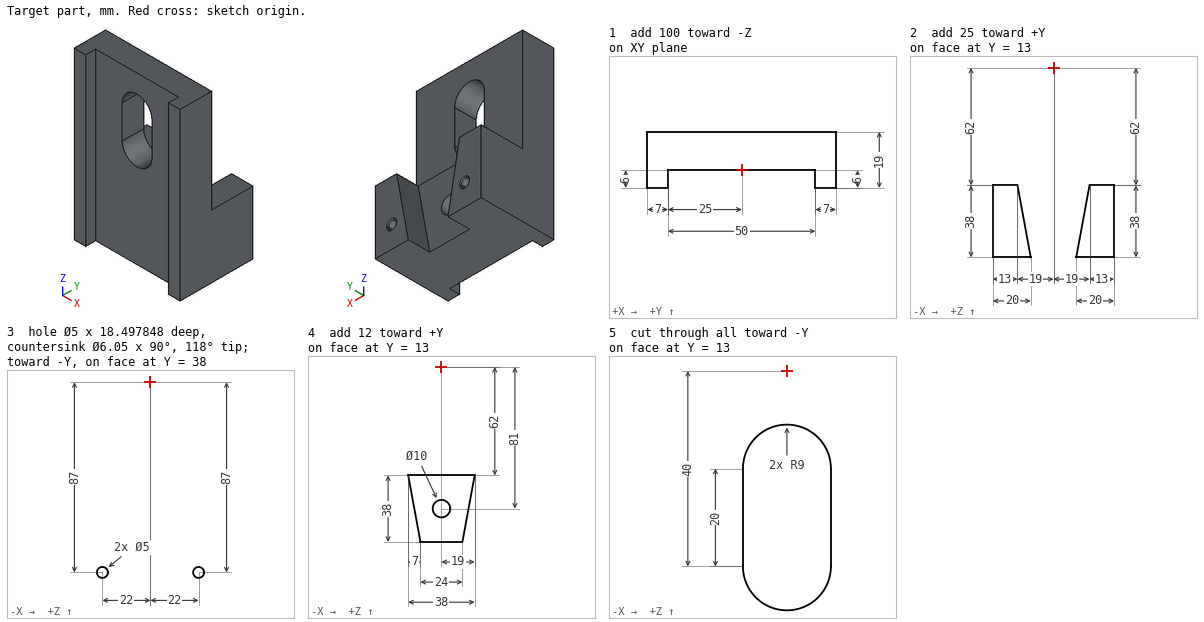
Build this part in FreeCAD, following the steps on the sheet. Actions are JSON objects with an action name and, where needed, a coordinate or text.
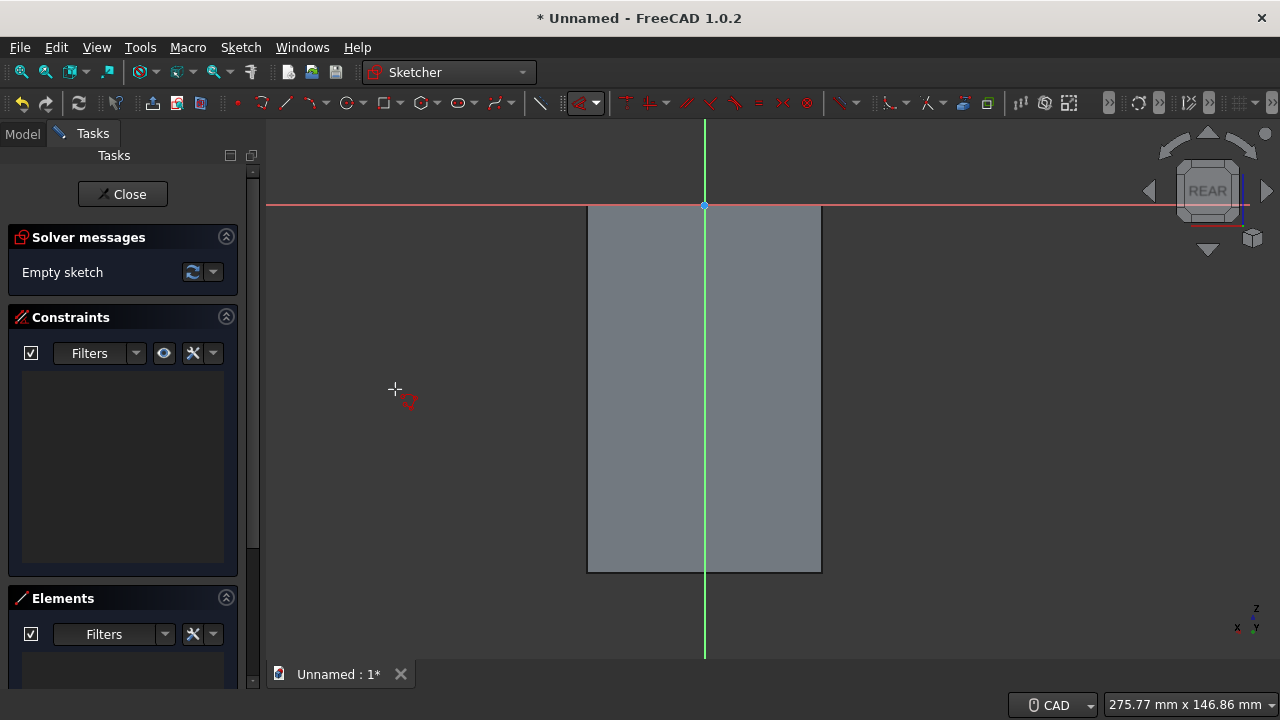
{"action": "left_click", "coordinate": [635, 433]}
{"action": "left_click", "coordinate": [587, 433]}
{"action": "left_click", "coordinate": [587, 573]}
{"action": "left_click", "coordinate": [660, 573]}
{"action": "left_click", "coordinate": [635, 434]}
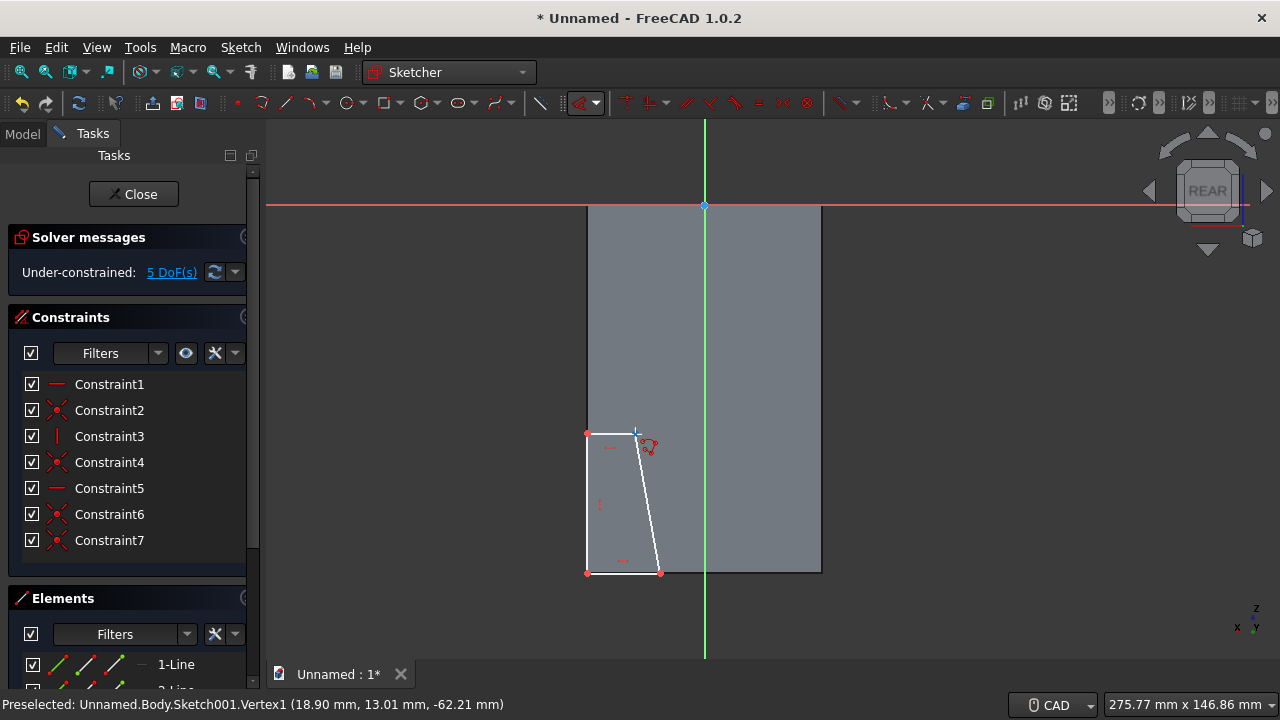
{"action": "left_click", "coordinate": [774, 433]}
{"action": "left_click", "coordinate": [749, 573]}
{"action": "left_click", "coordinate": [822, 573]}
{"action": "left_click", "coordinate": [822, 433]}
{"action": "left_click", "coordinate": [774, 434]}
{"action": "key", "text": "Escape"}
{"action": "key", "text": "Escape"}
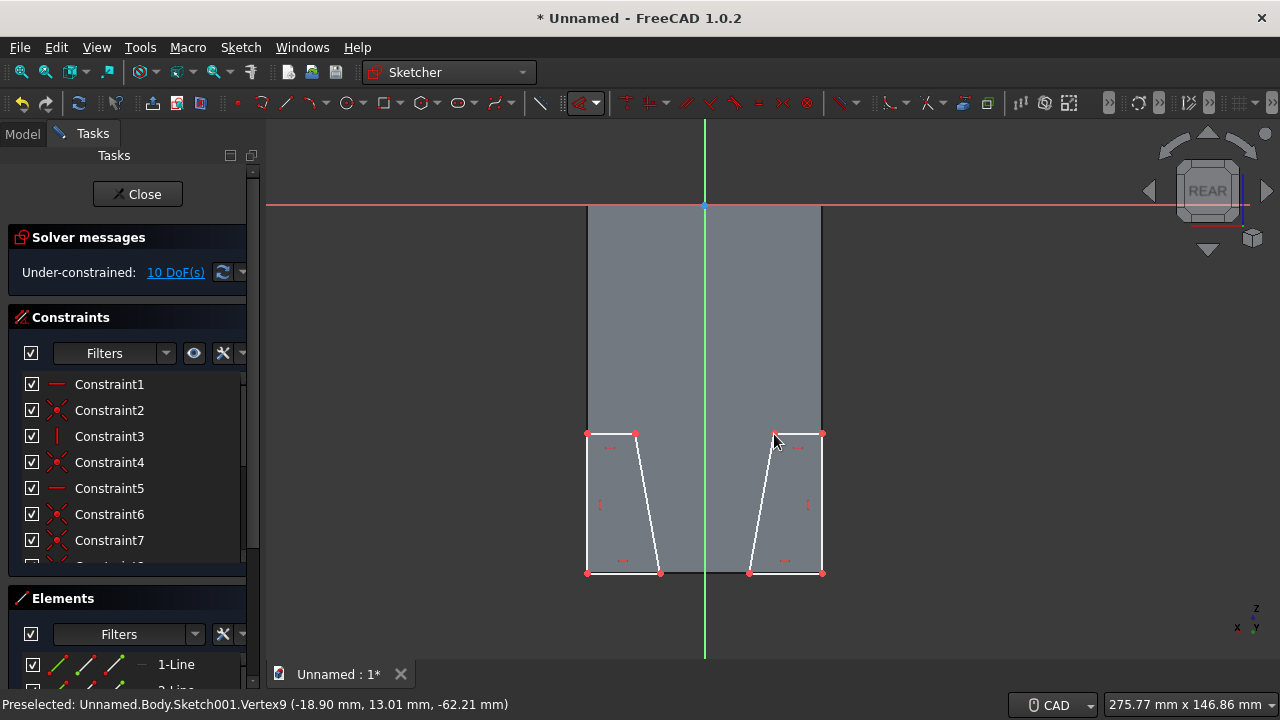
{"action": "left_click", "coordinate": [580, 104]}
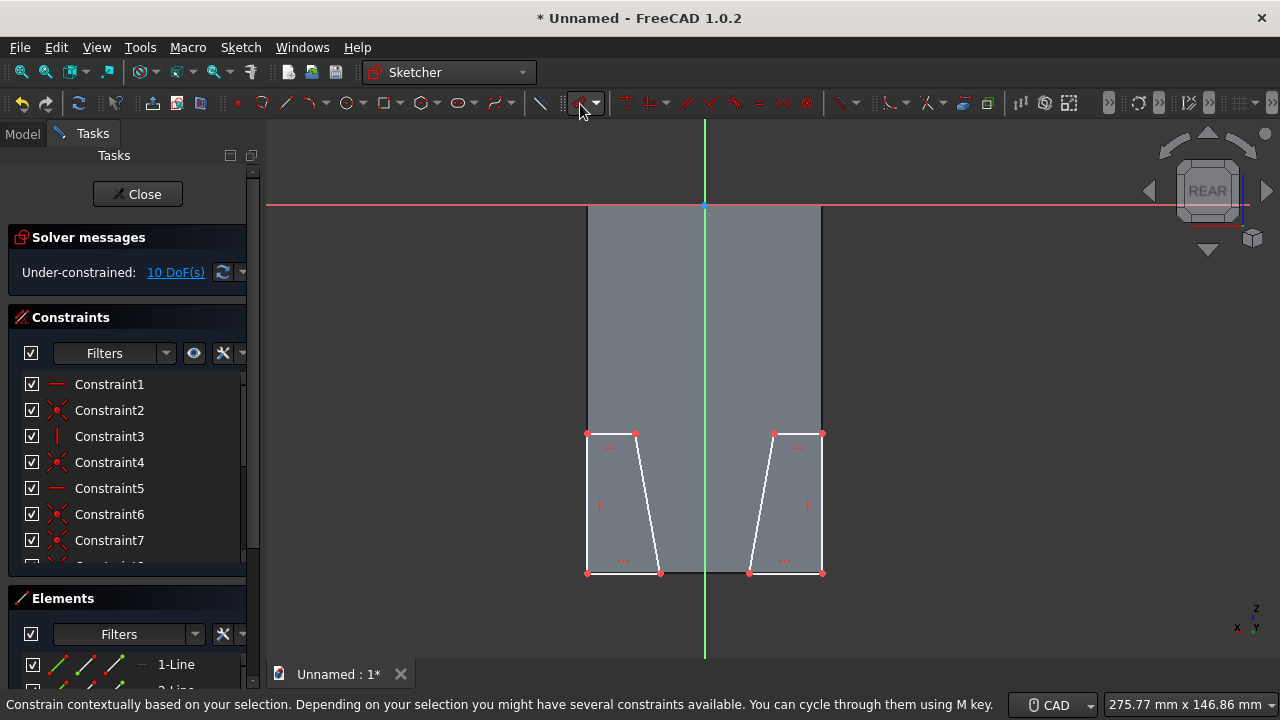
{"action": "left_click", "coordinate": [621, 434]}
{"action": "left_click", "coordinate": [611, 468]}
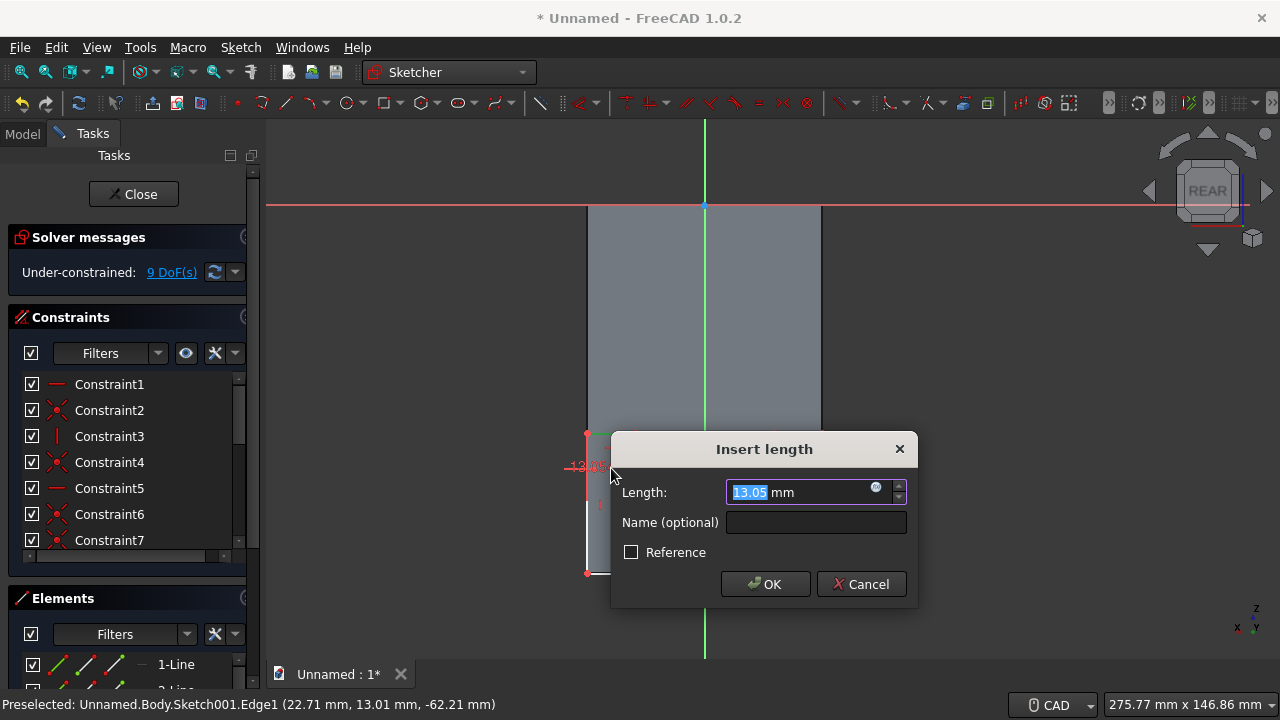
{"action": "type", "text": "13"}
{"action": "key", "text": "Return"}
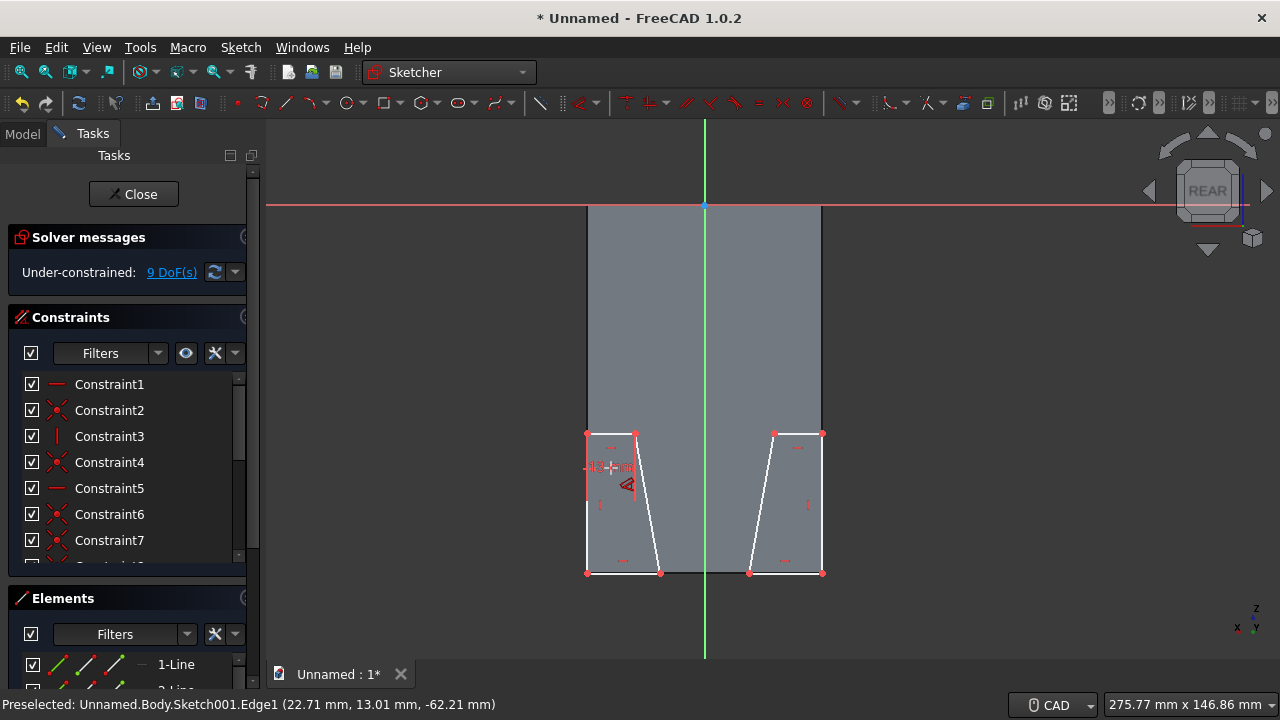
{"action": "left_click", "coordinate": [587, 476]}
{"action": "left_click", "coordinate": [553, 504]}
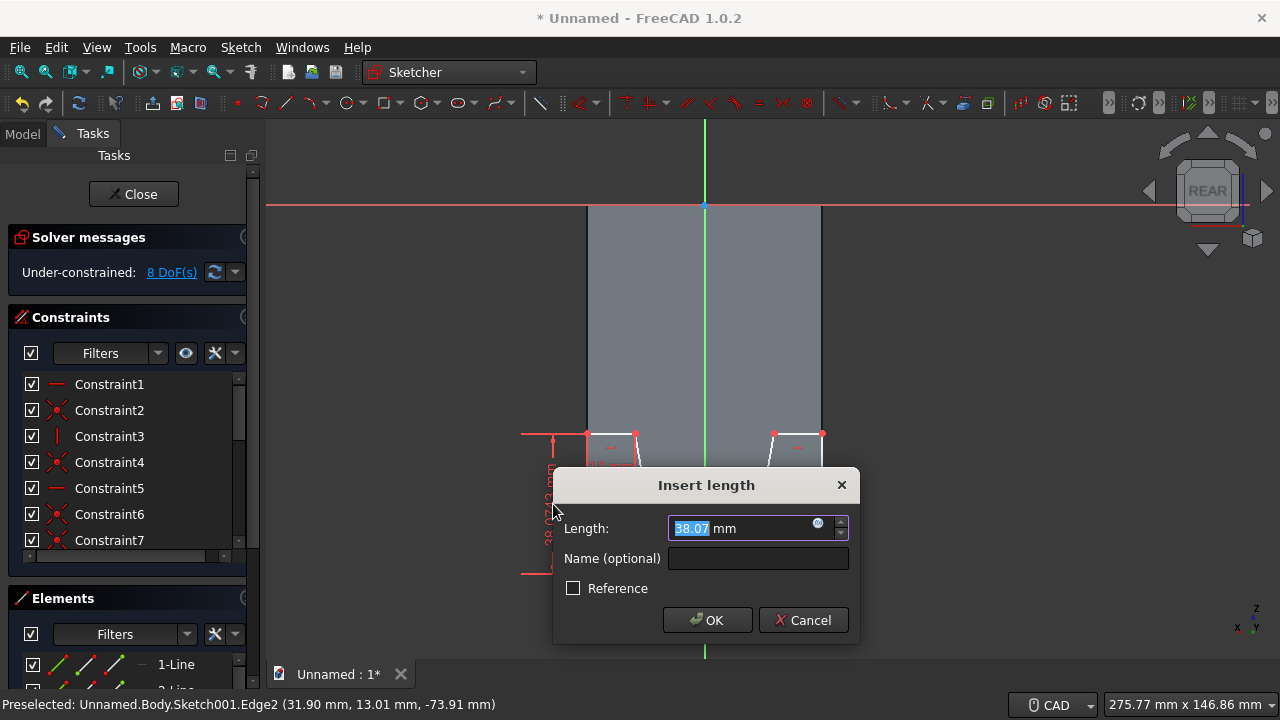
{"action": "type", "text": "38"}
{"action": "key", "text": "Return"}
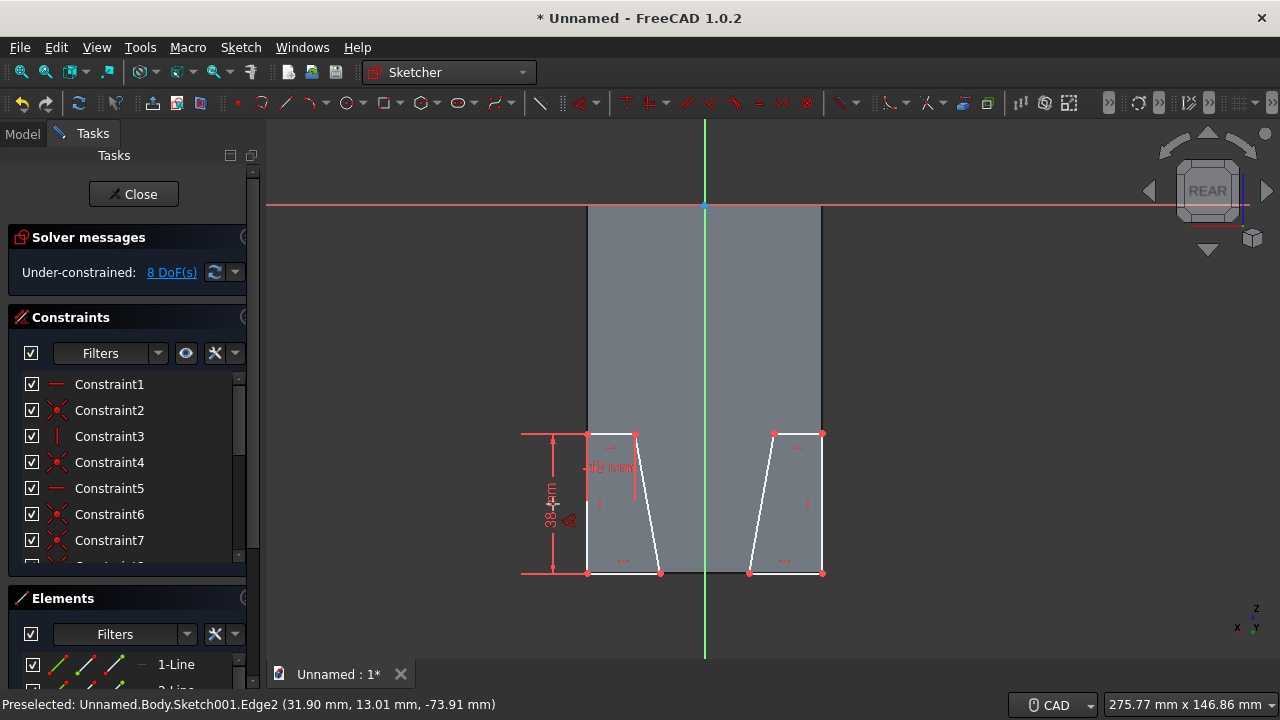
{"action": "left_click", "coordinate": [609, 574]}
{"action": "left_click", "coordinate": [624, 608]}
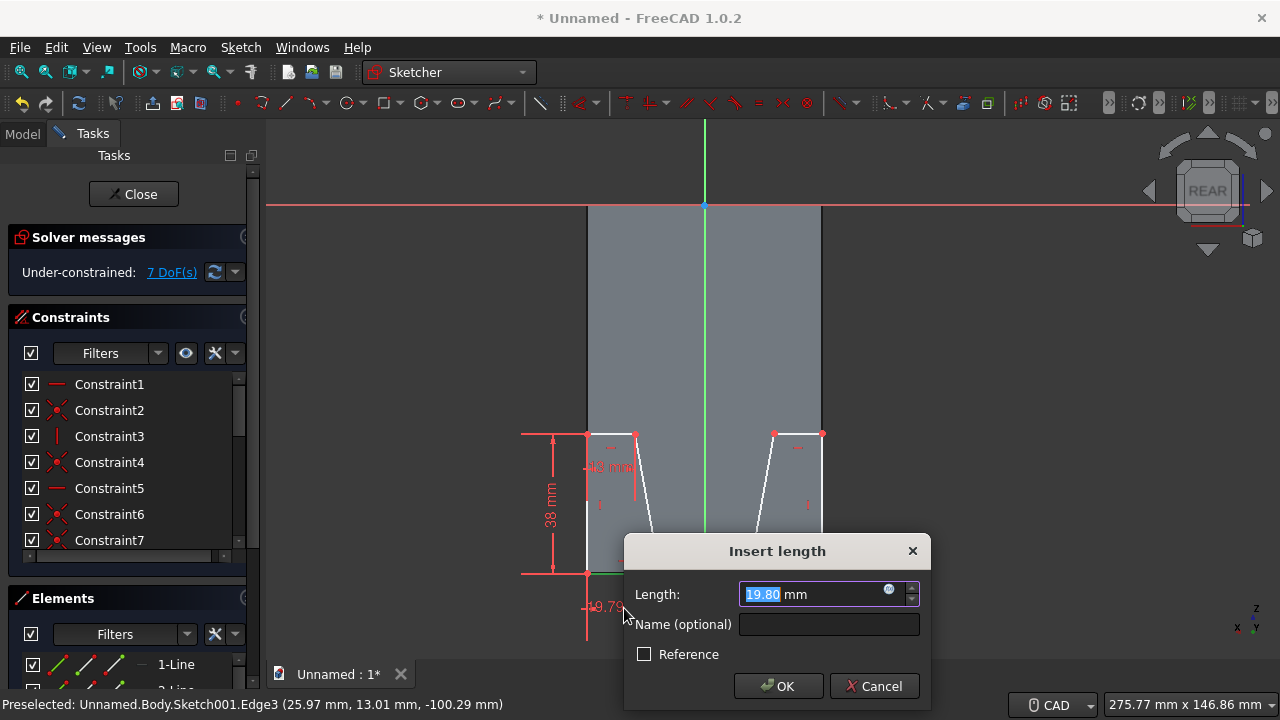
{"action": "type", "text": "20"}
{"action": "key", "text": "Return"}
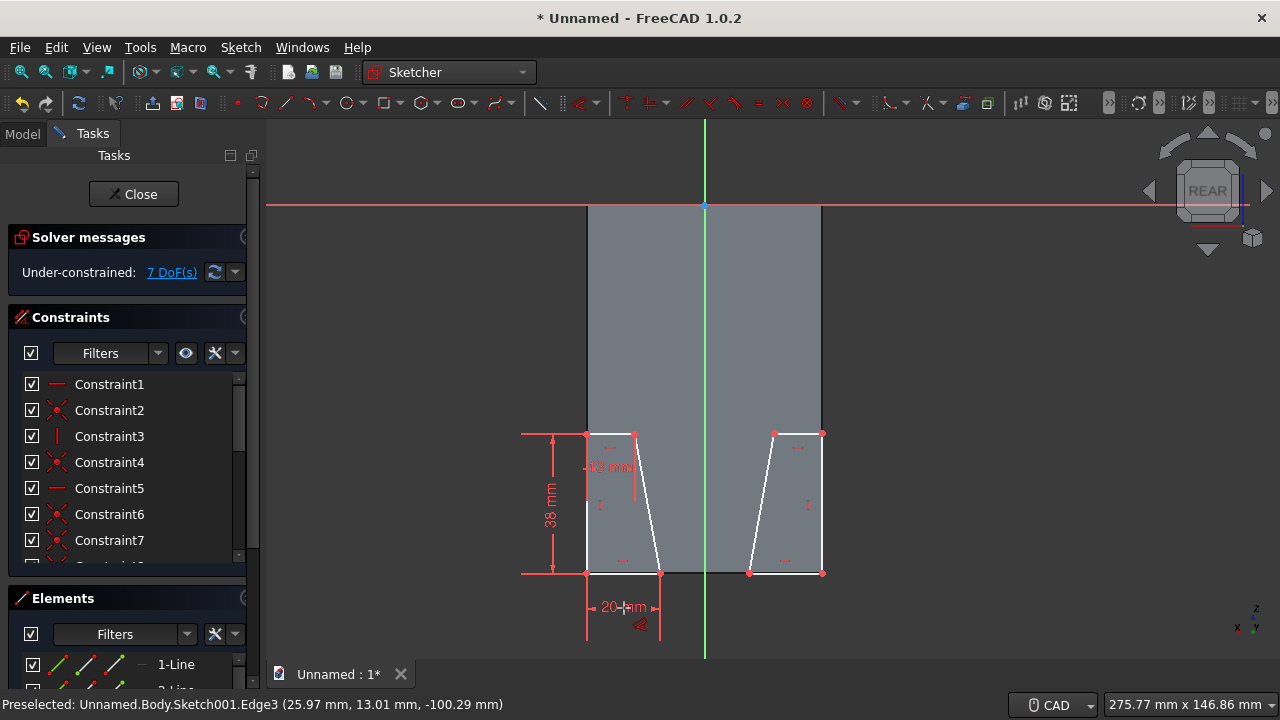
{"action": "left_click", "coordinate": [771, 574]}
{"action": "left_click", "coordinate": [785, 608]}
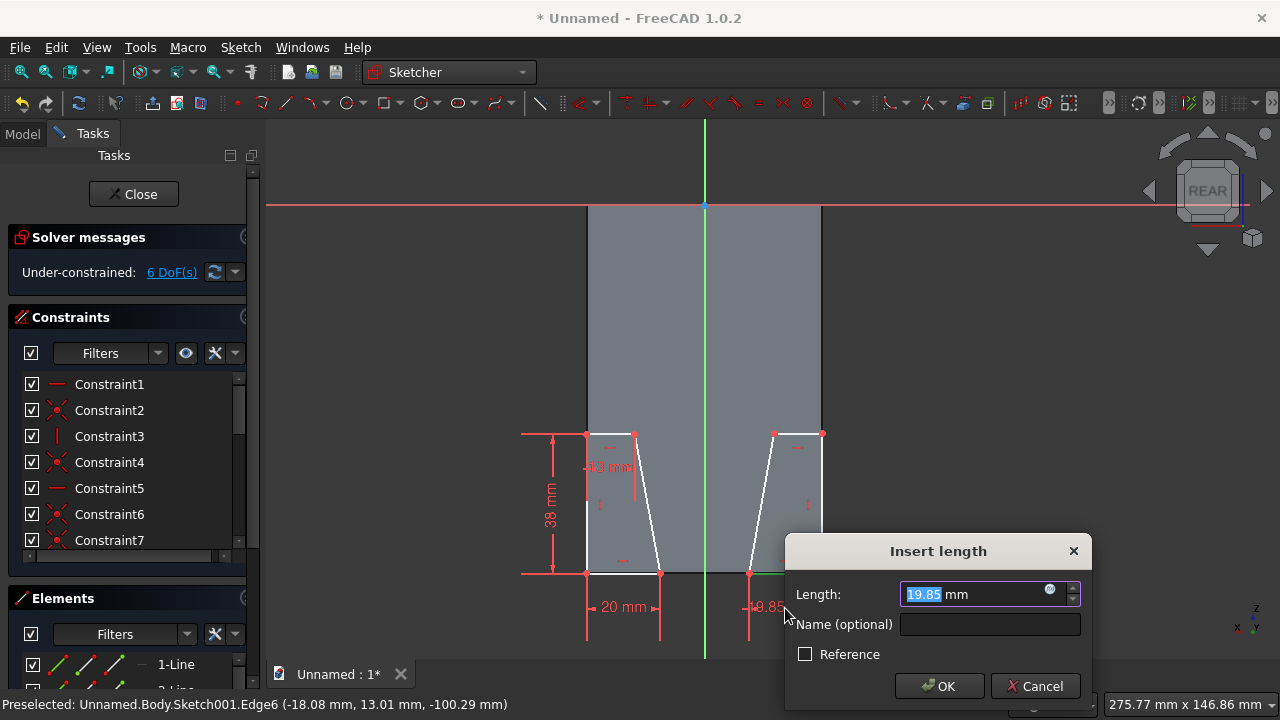
{"action": "type", "text": "20"}
{"action": "key", "text": "Return"}